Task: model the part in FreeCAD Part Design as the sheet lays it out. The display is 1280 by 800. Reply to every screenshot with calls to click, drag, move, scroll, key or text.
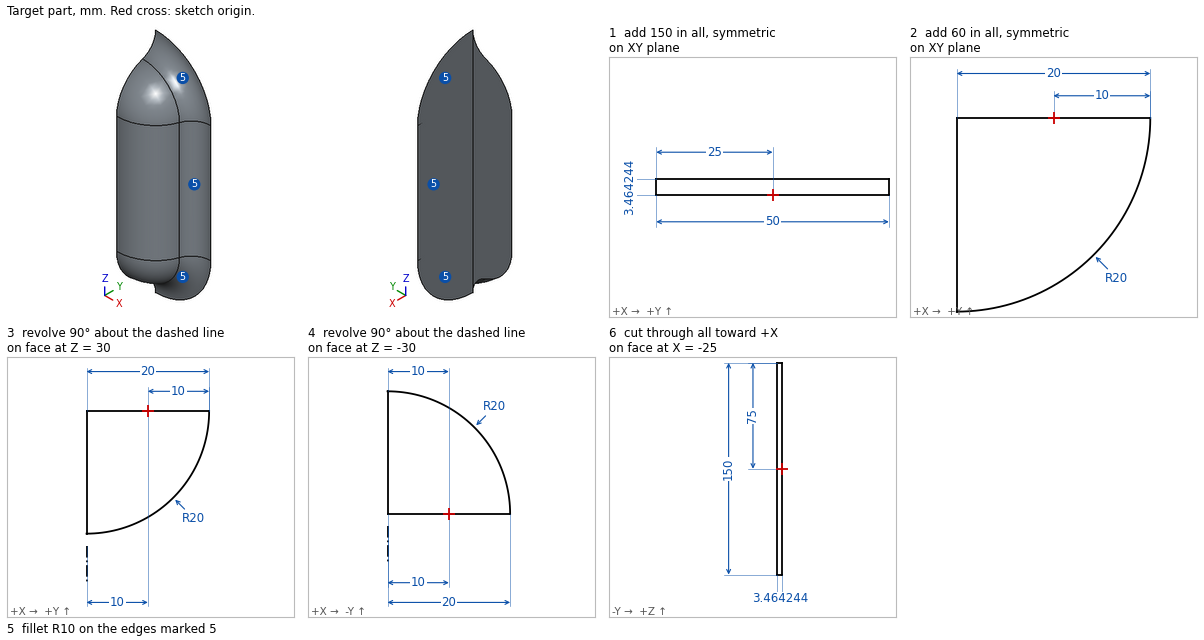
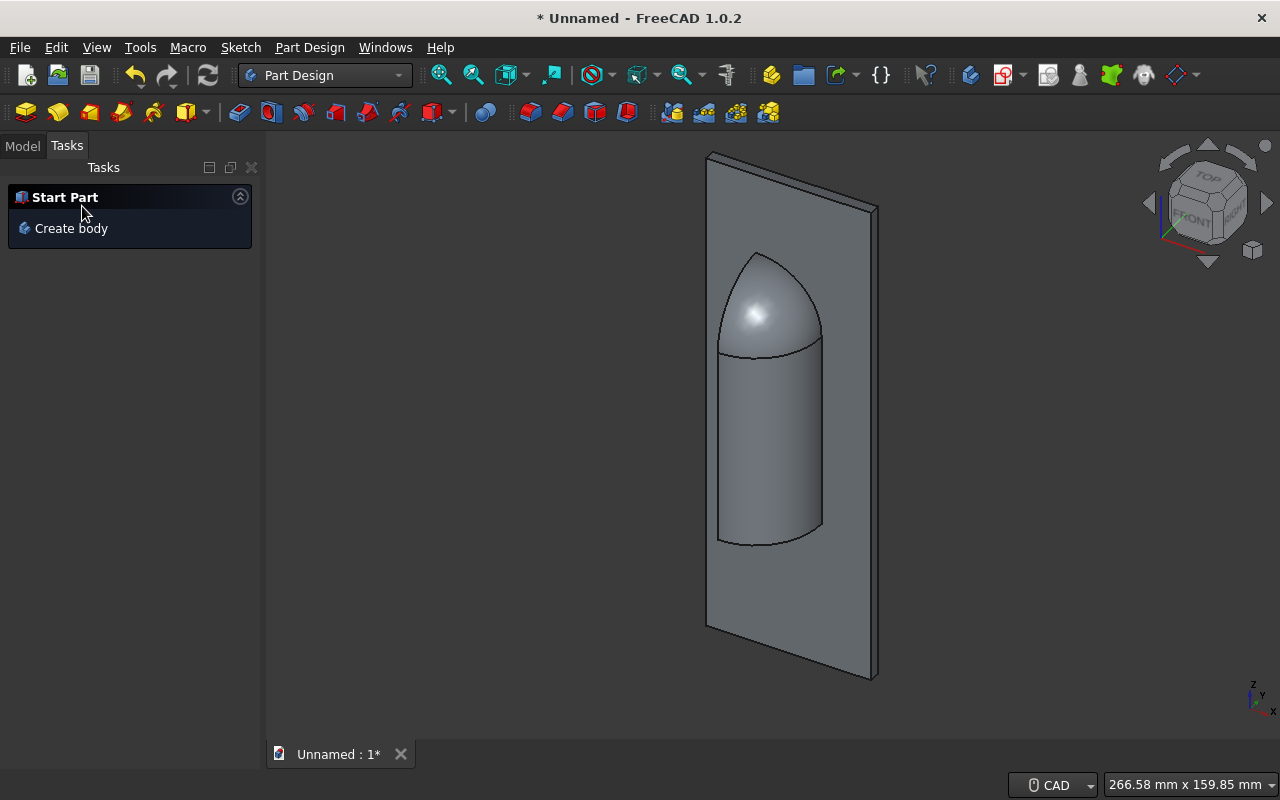
key(5)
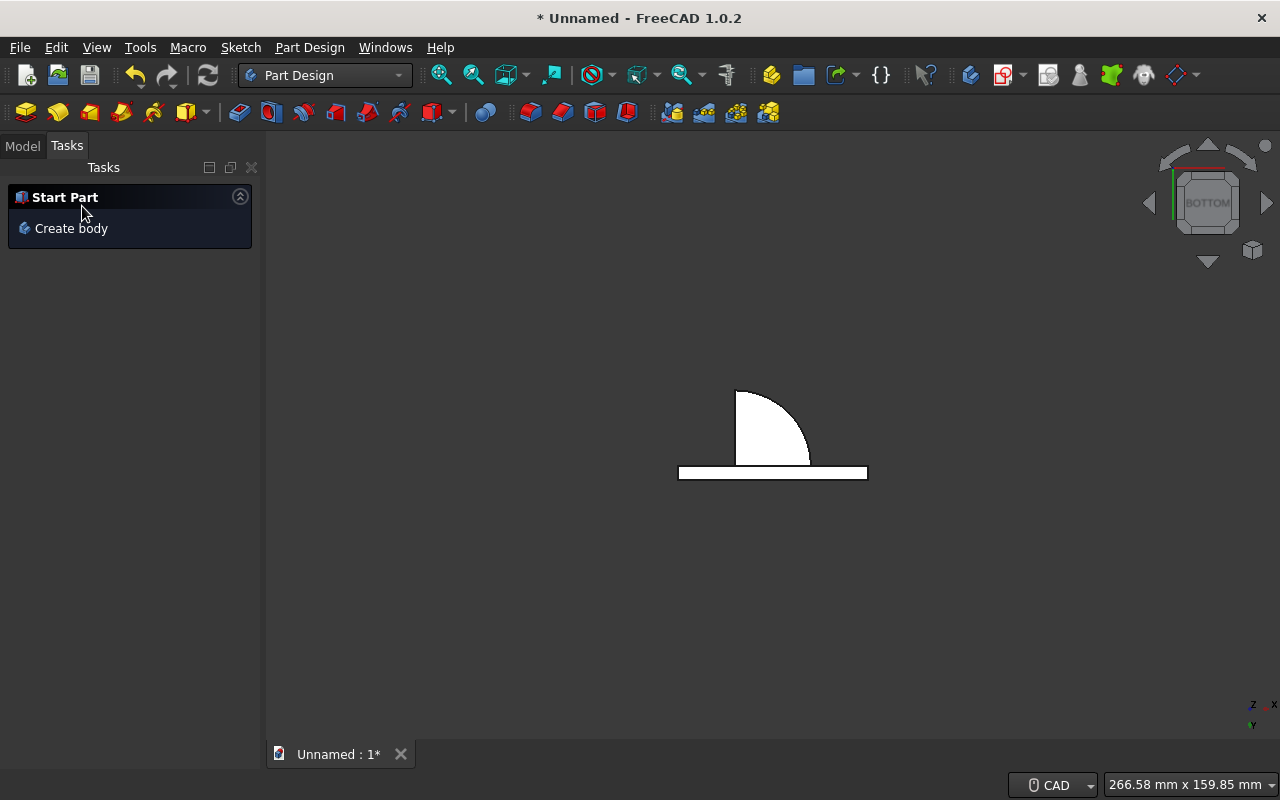
click(442, 76)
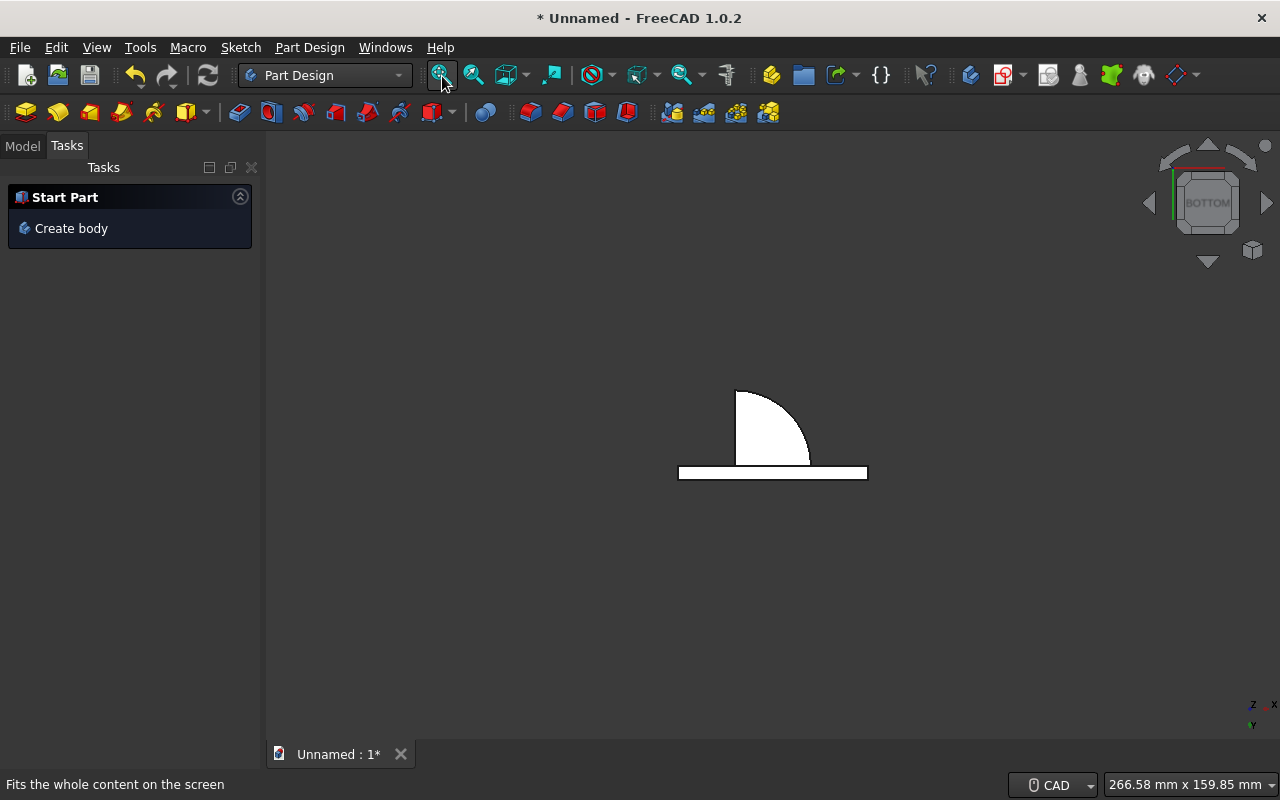
click(762, 427)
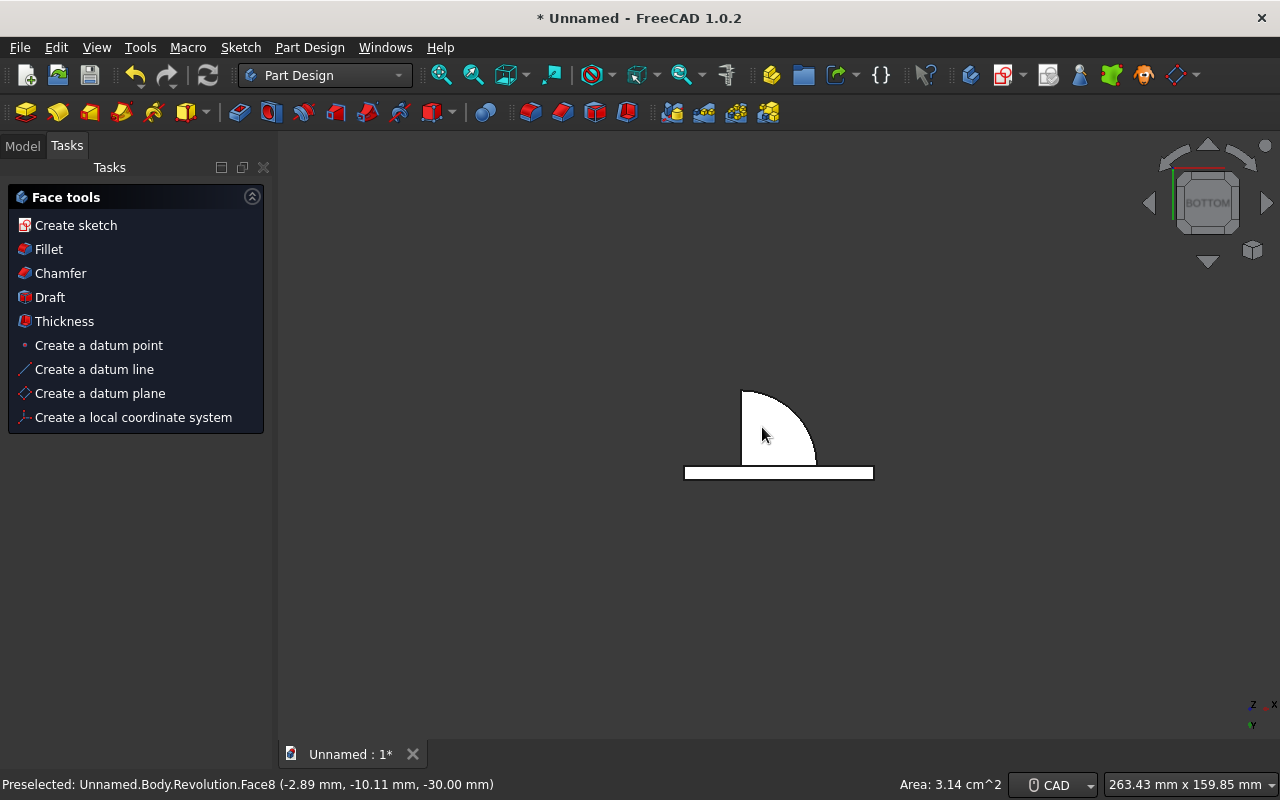
click(1004, 76)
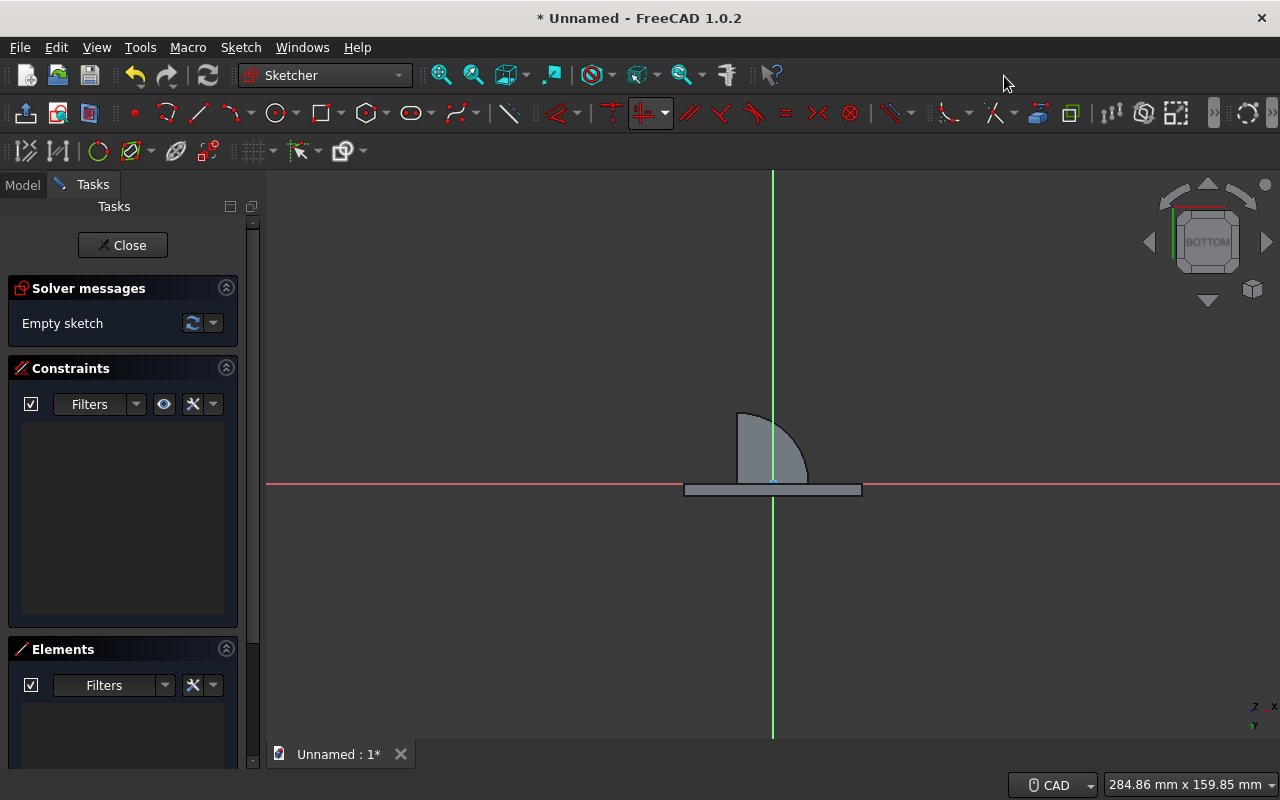
scroll(803, 466, up, 6)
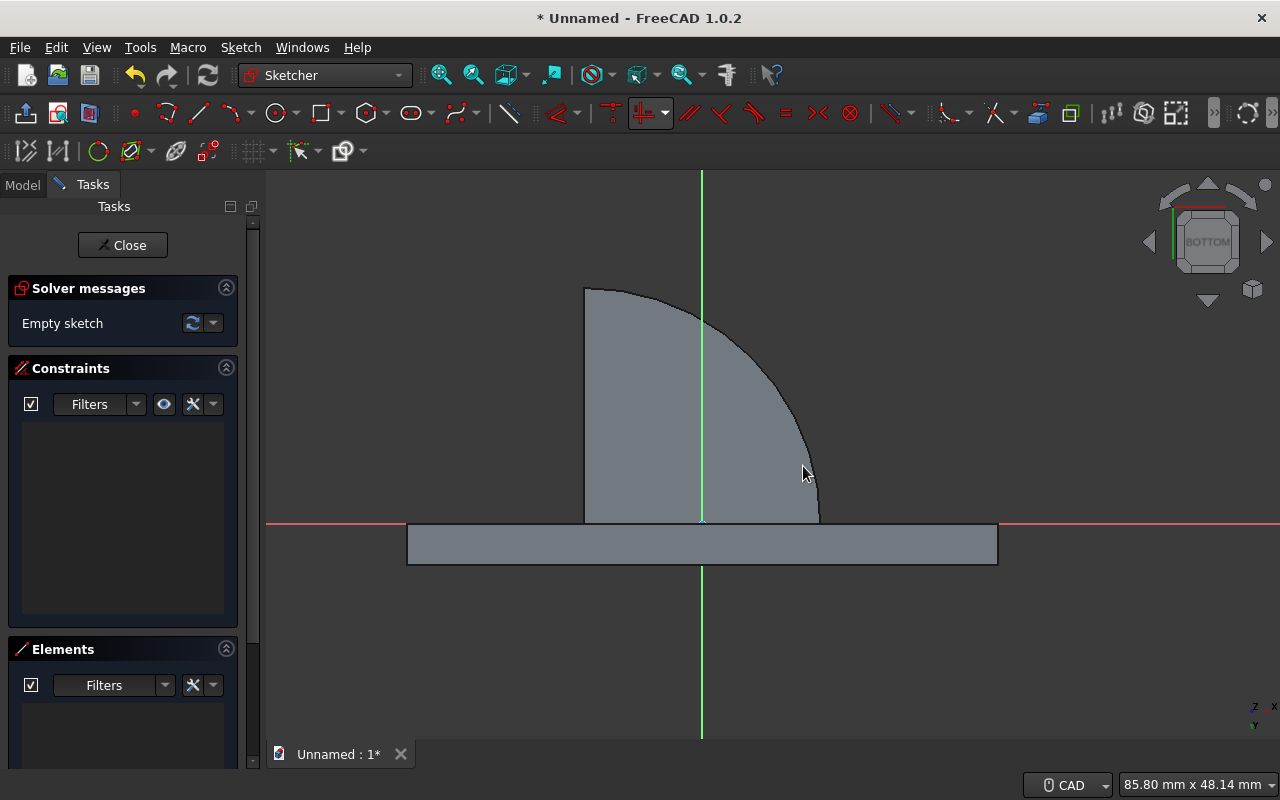
click(168, 114)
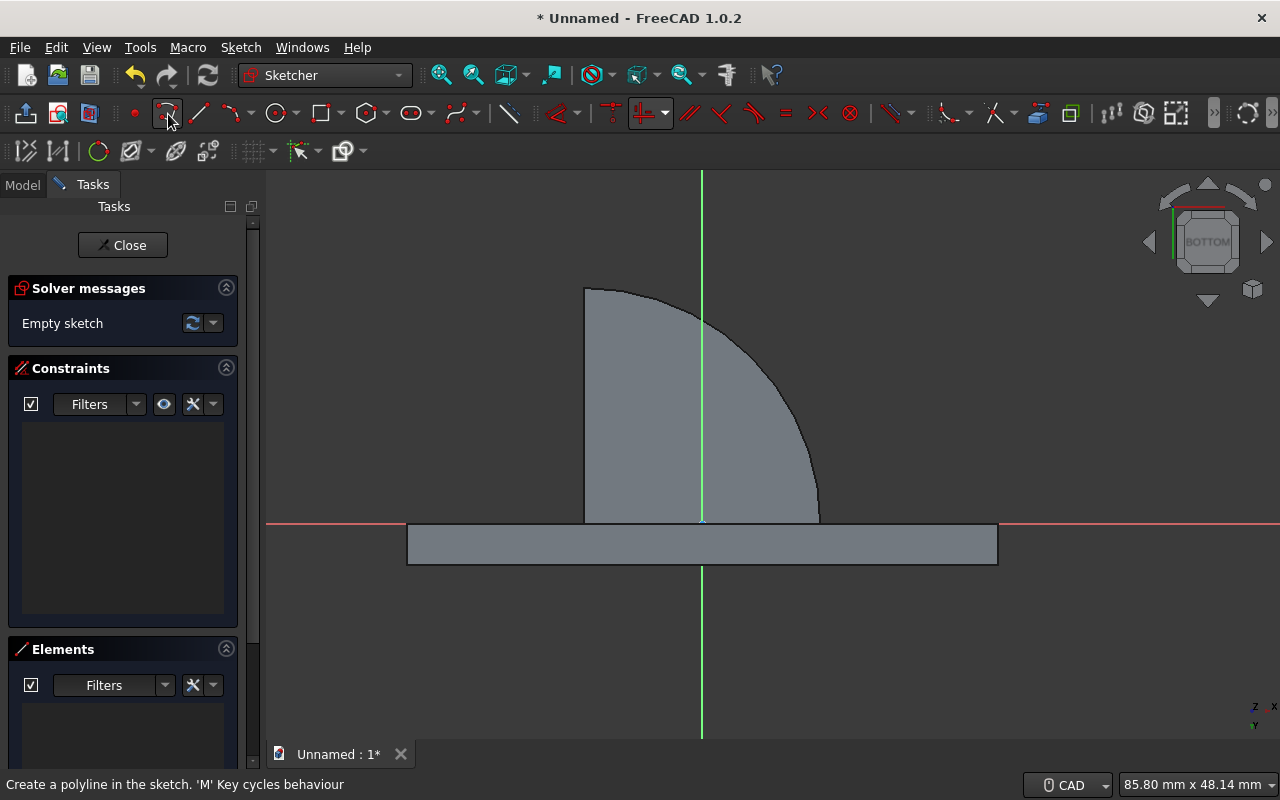
click(584, 288)
click(584, 524)
click(820, 515)
right_click(820, 515)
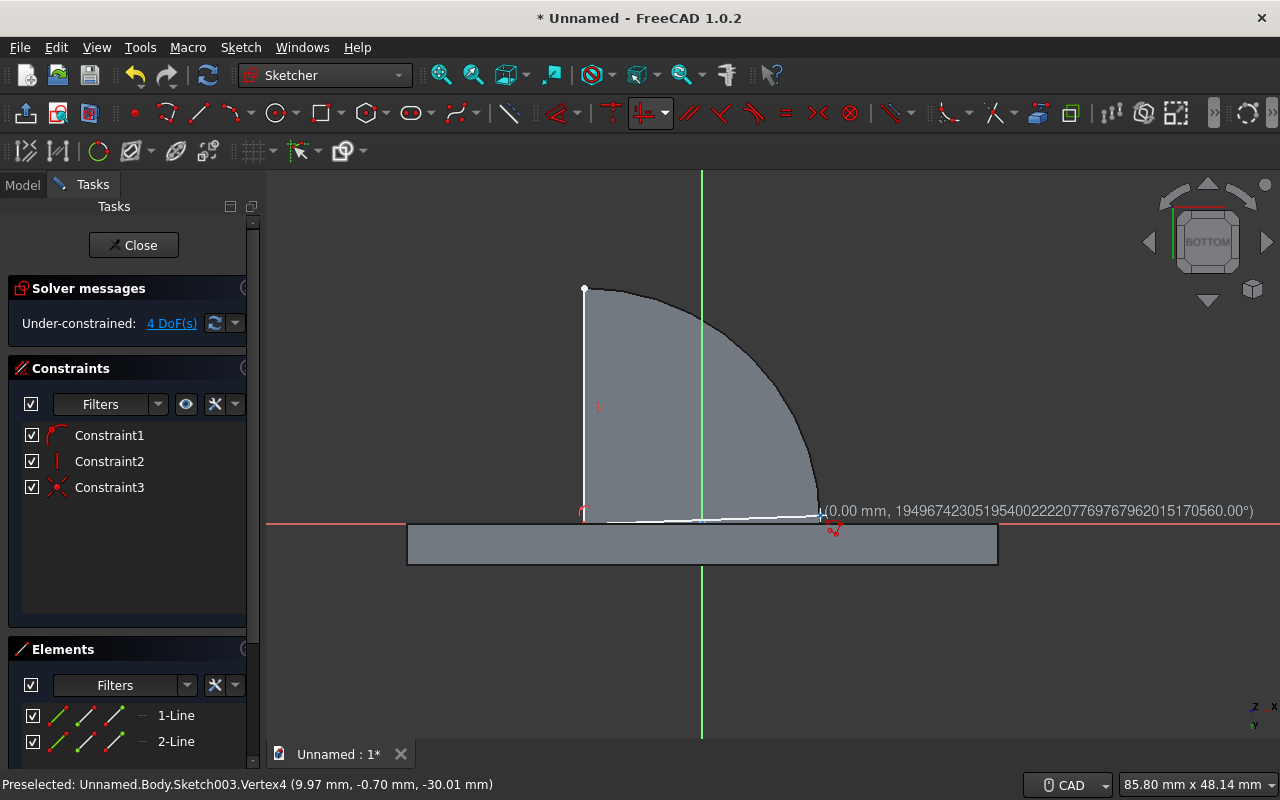
click(232, 114)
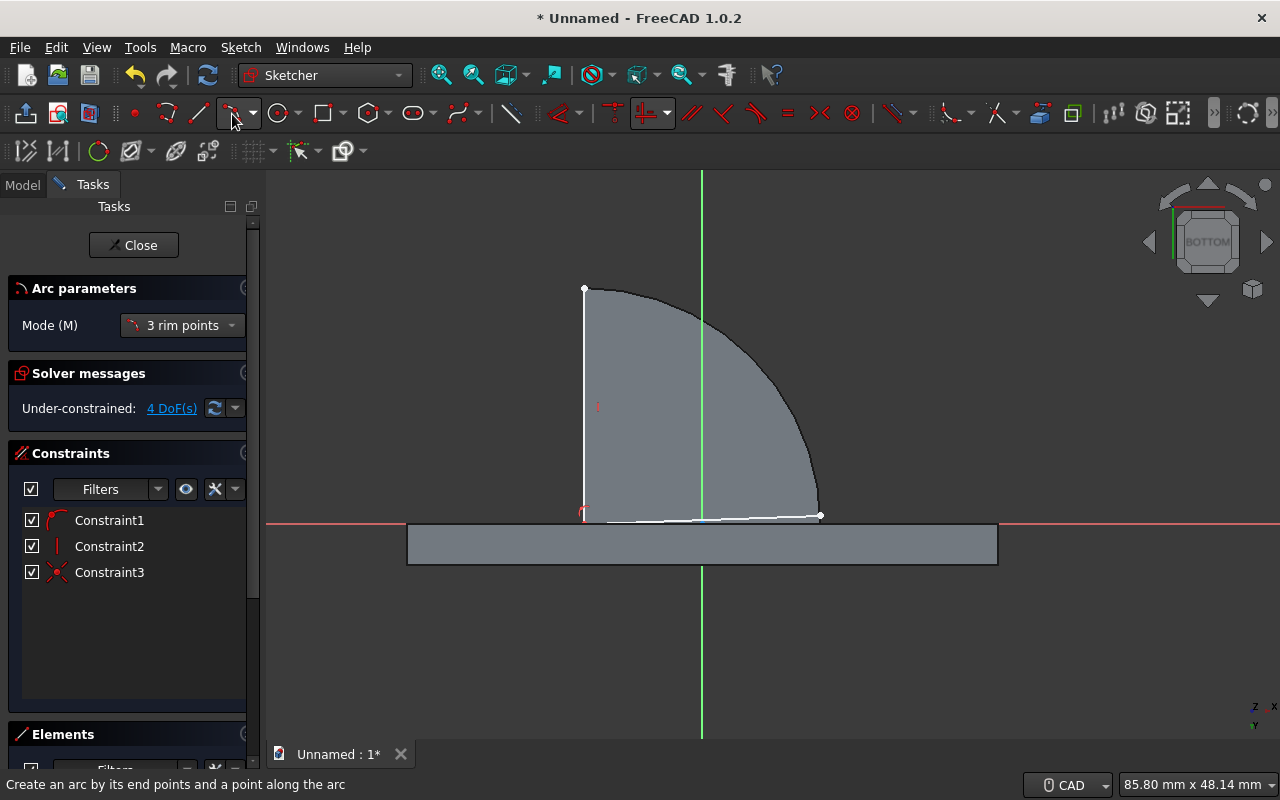
click(820, 516)
click(584, 289)
click(751, 357)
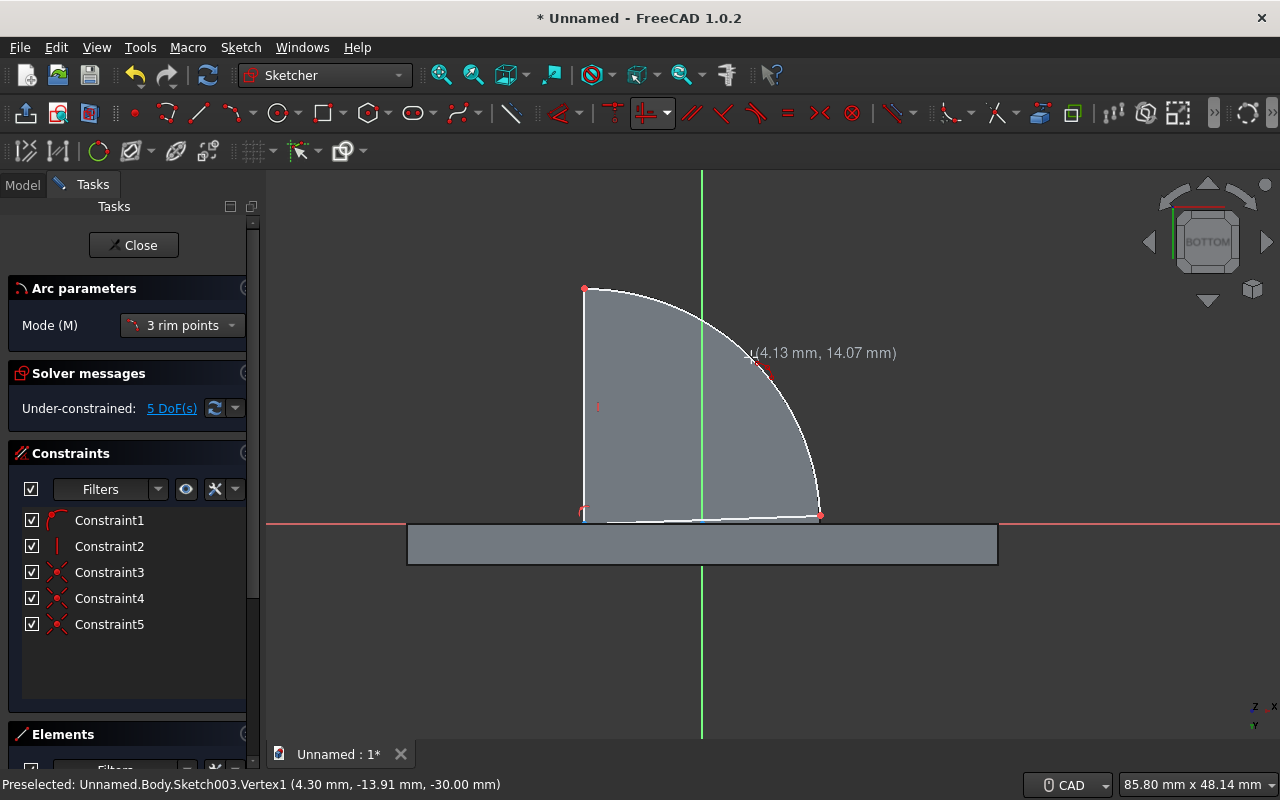
click(200, 114)